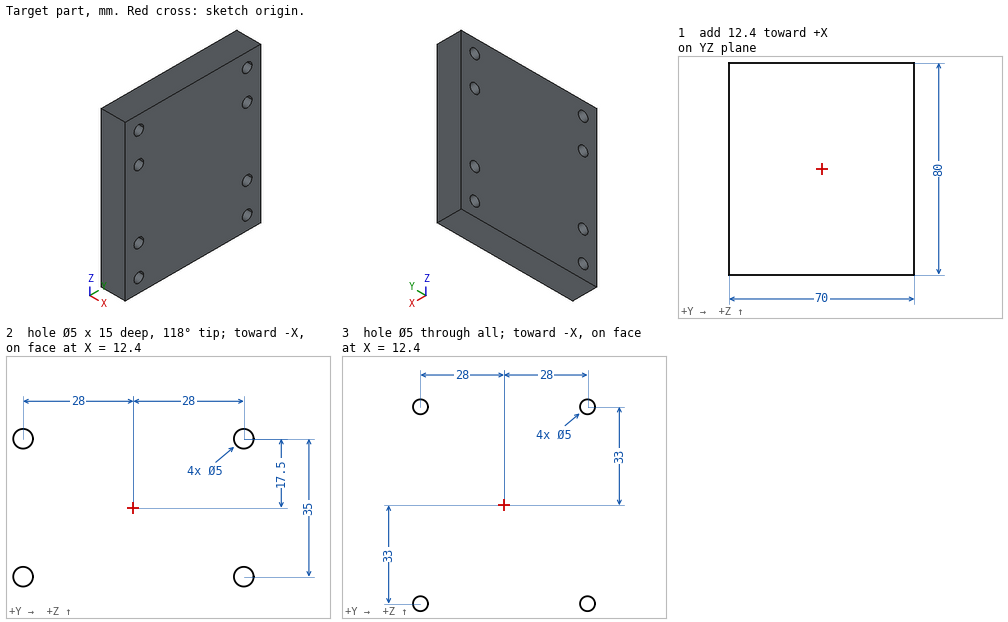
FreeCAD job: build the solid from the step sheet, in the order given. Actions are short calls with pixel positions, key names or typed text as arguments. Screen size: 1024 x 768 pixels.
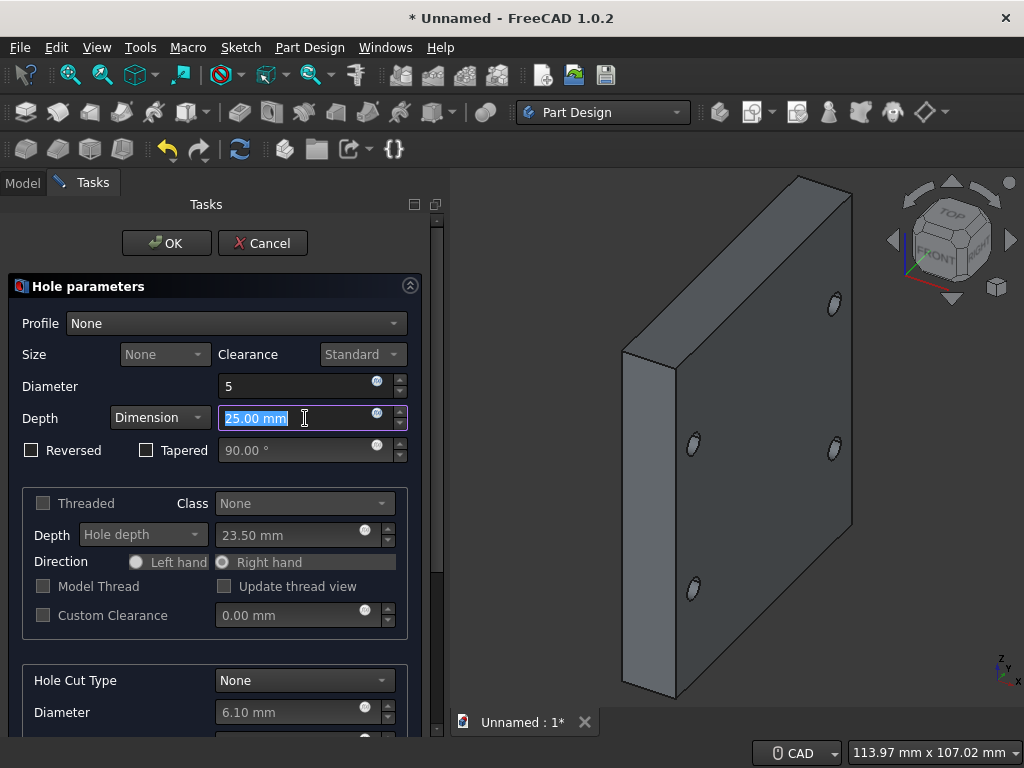
text(15)
key(Tab)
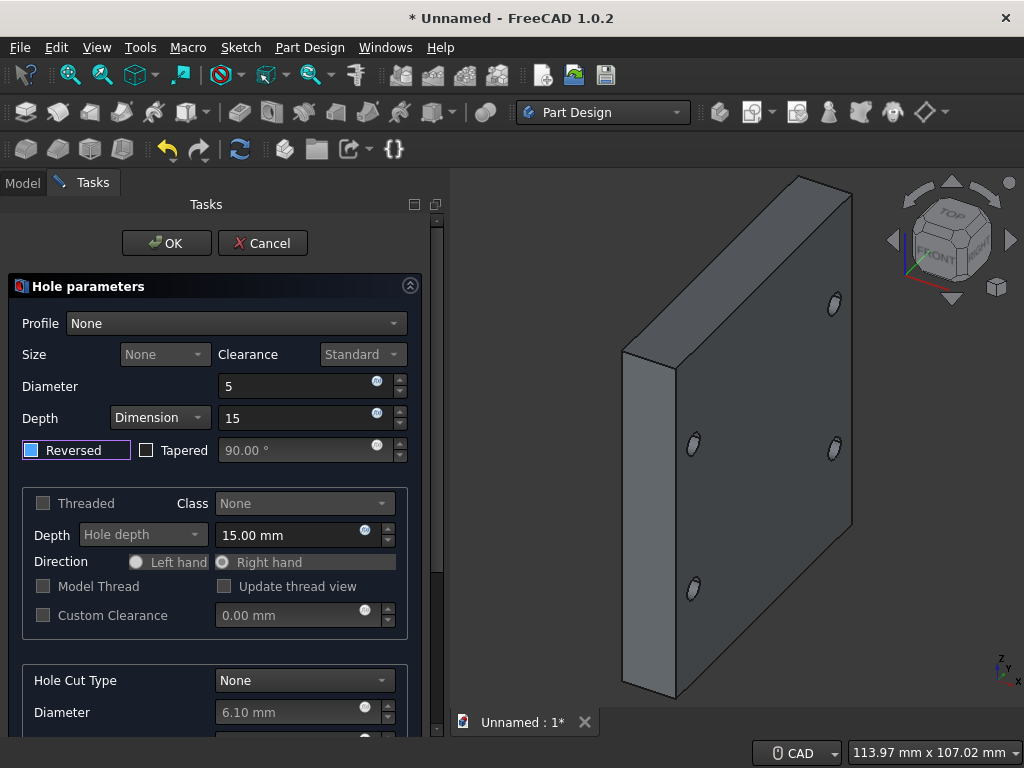
click(167, 243)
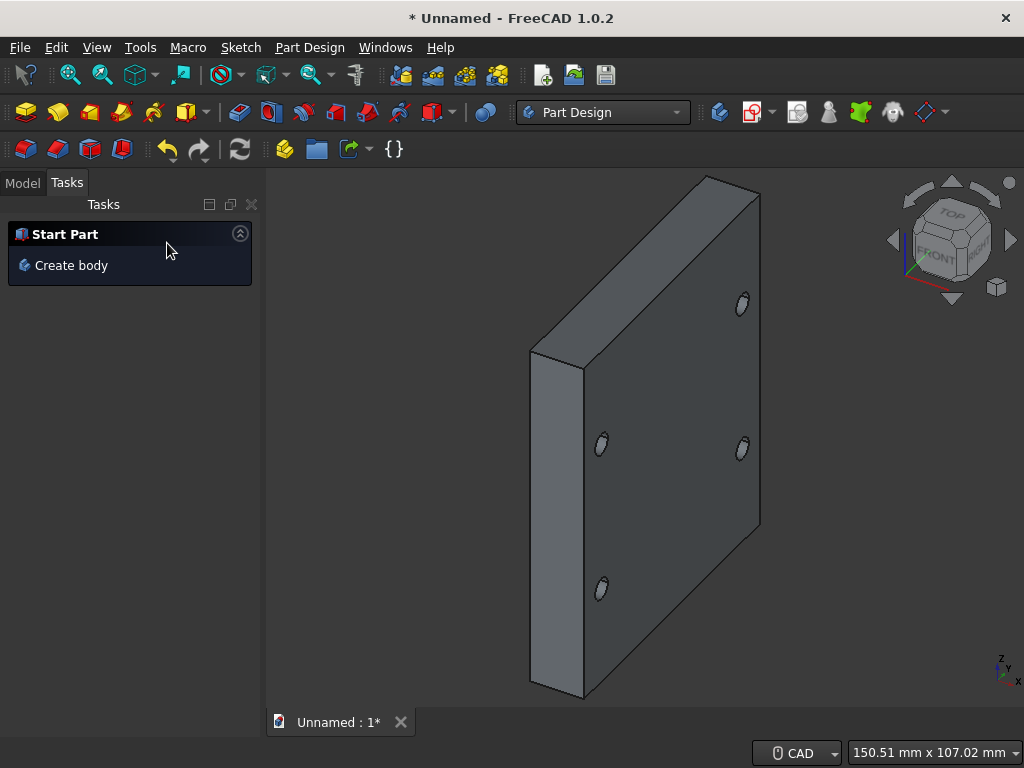
click(672, 445)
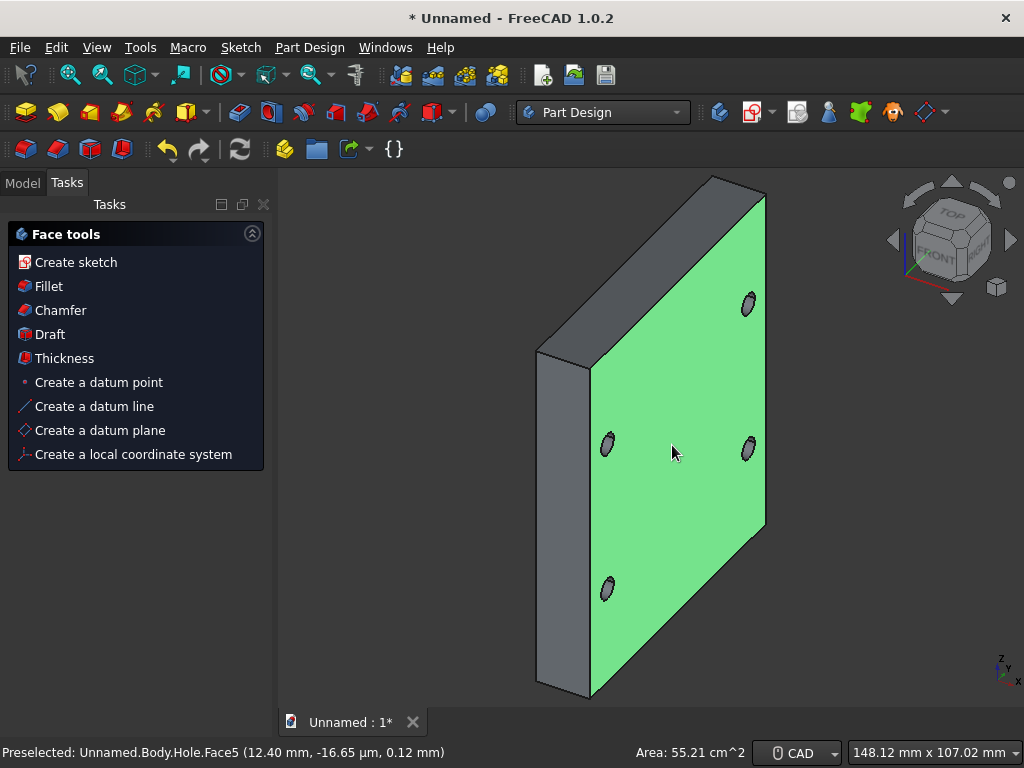
click(752, 112)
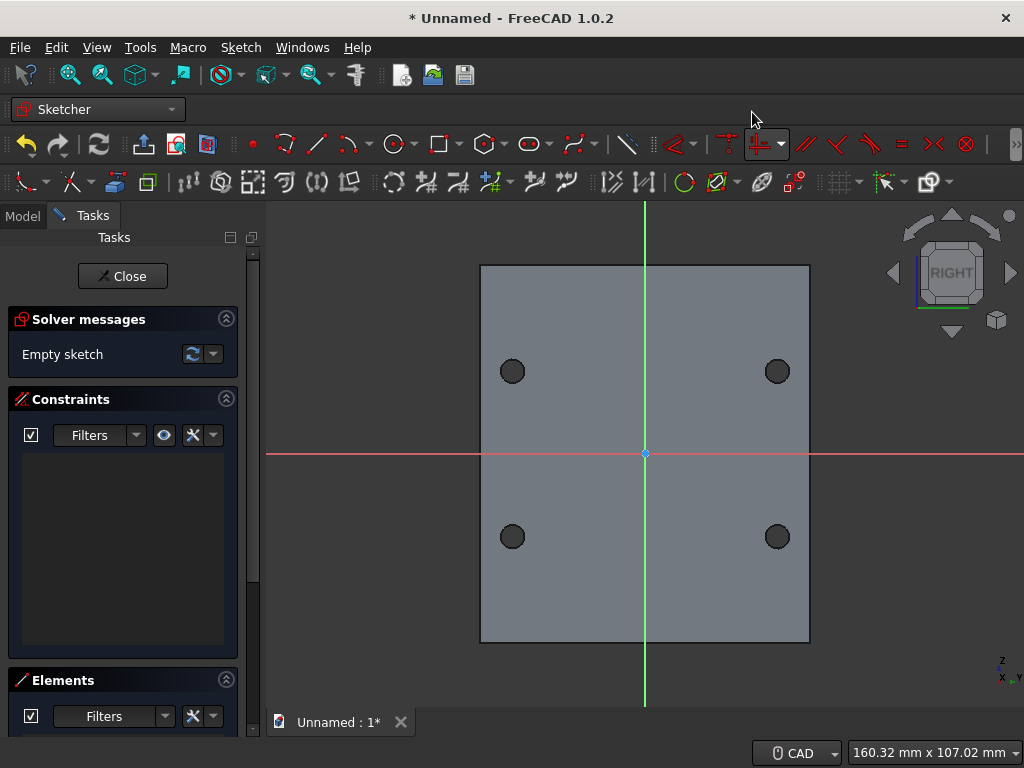
key(g)
key(c)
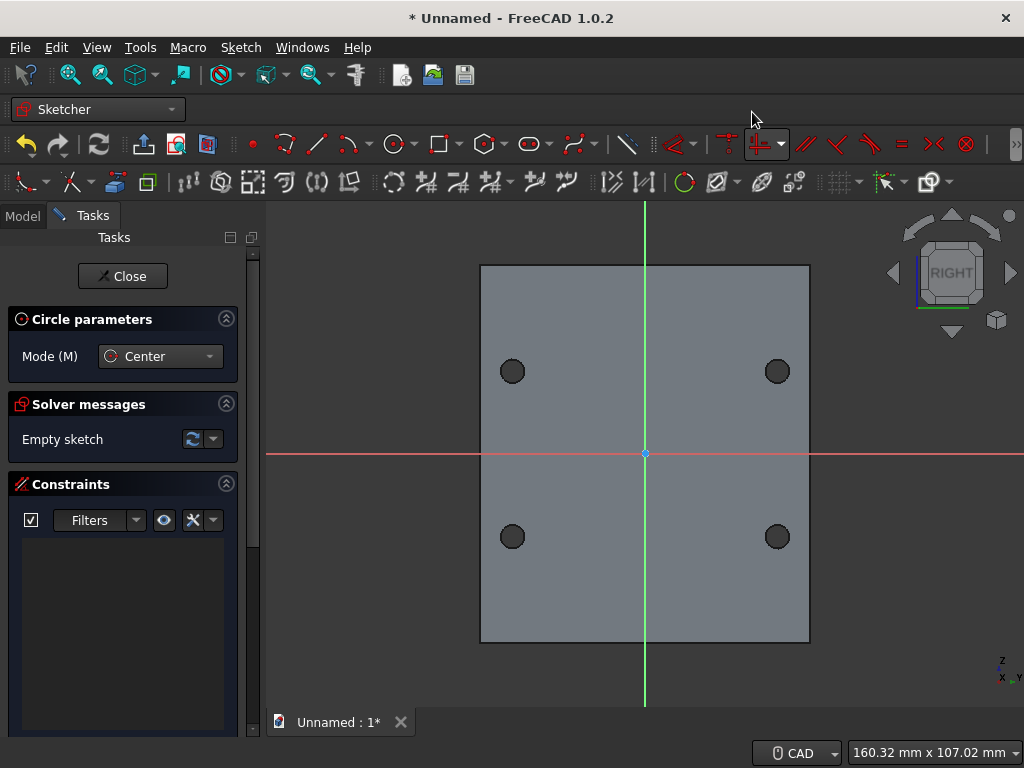
scroll(777, 298, up, 4)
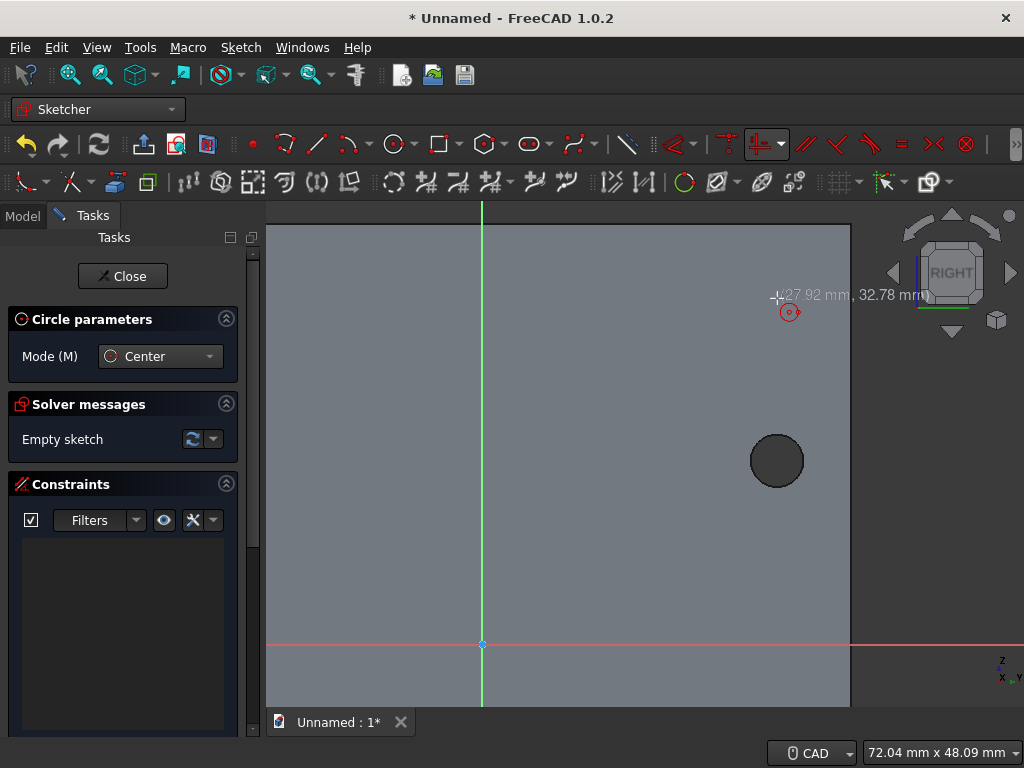
click(777, 298)
move(796, 279)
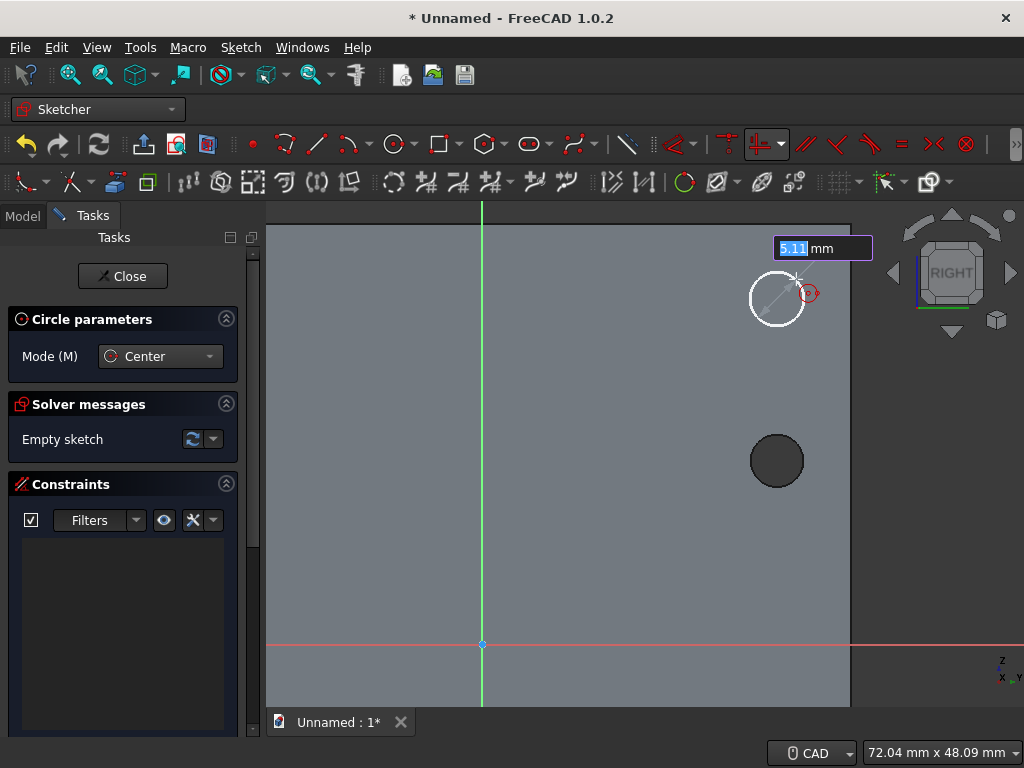
text(5)
key(Return)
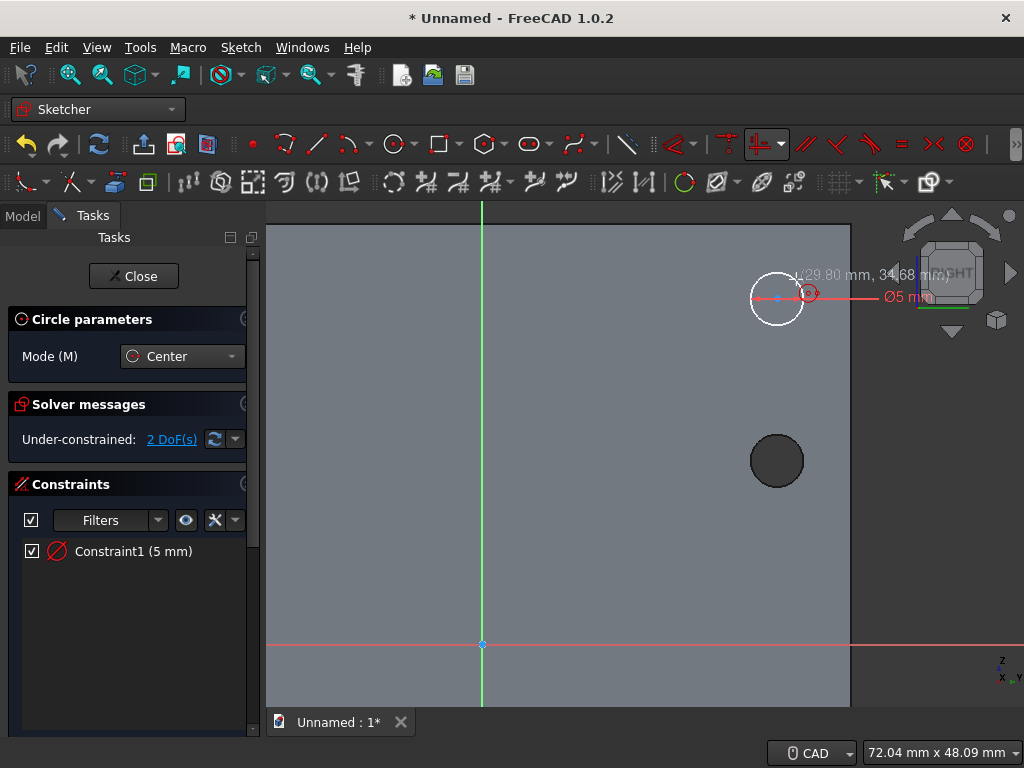
scroll(653, 298, down, 4)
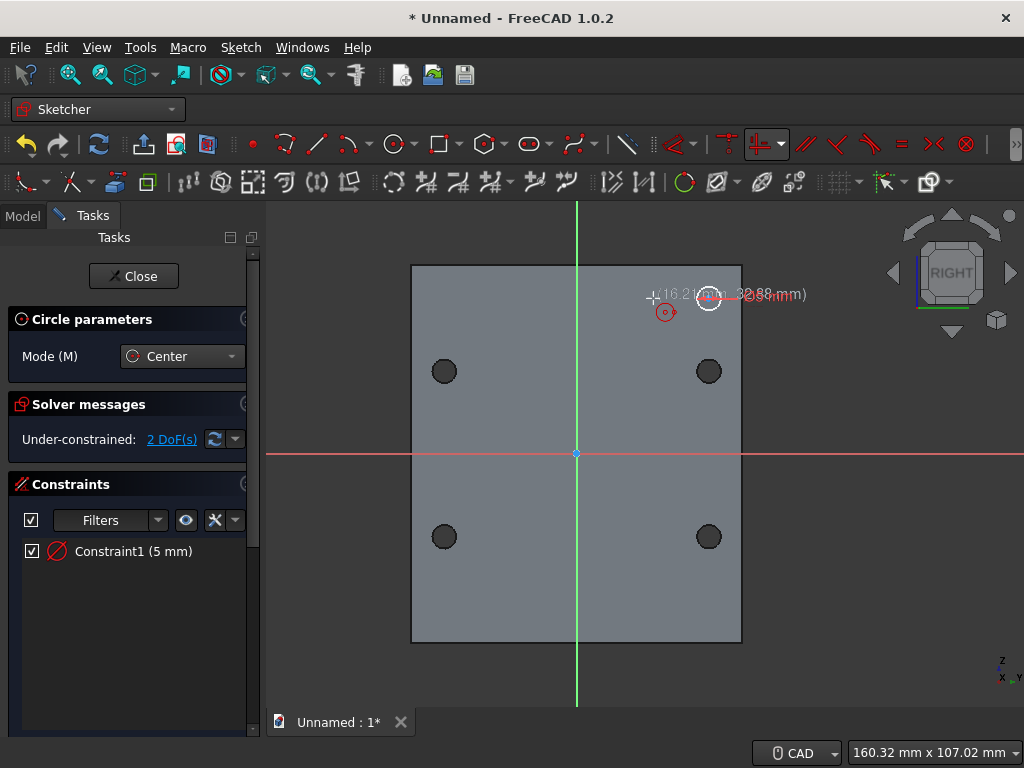
scroll(444, 298, up, 4)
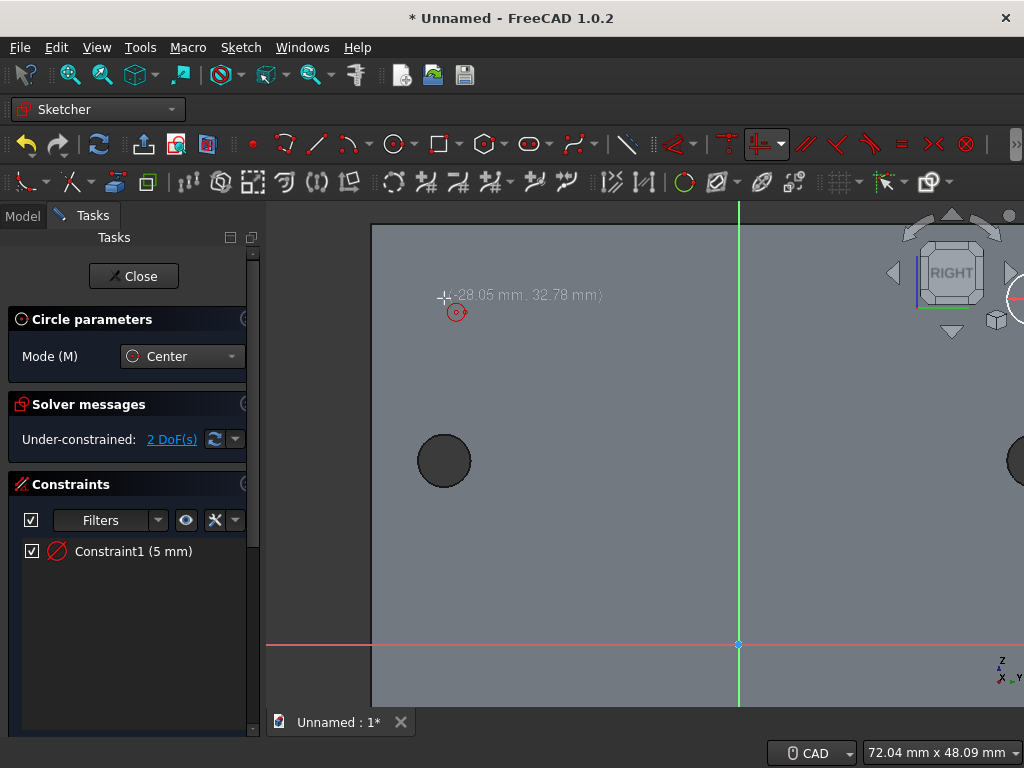
click(444, 298)
move(463, 279)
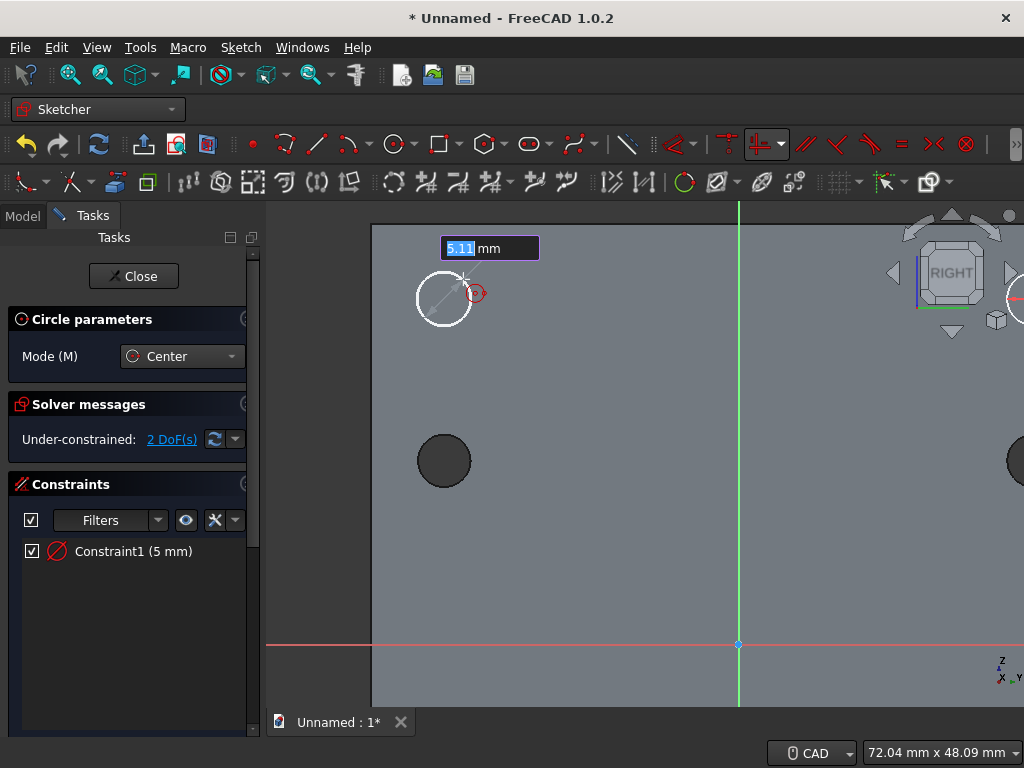
text(5)
key(Return)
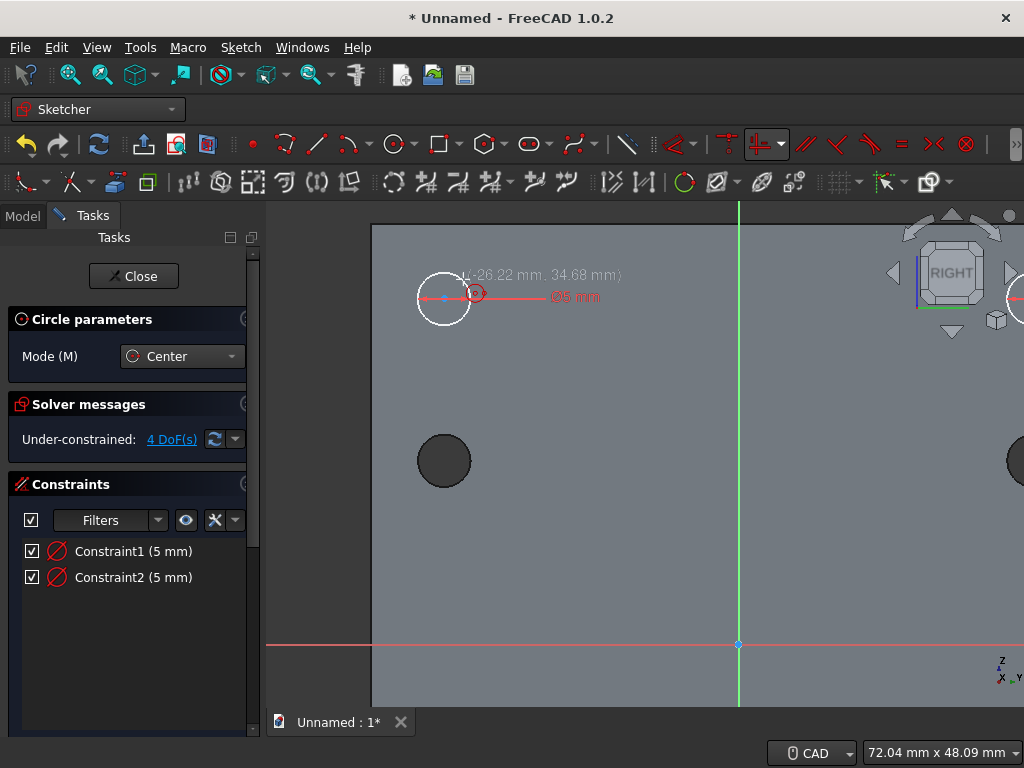
scroll(444, 298, down, 4)